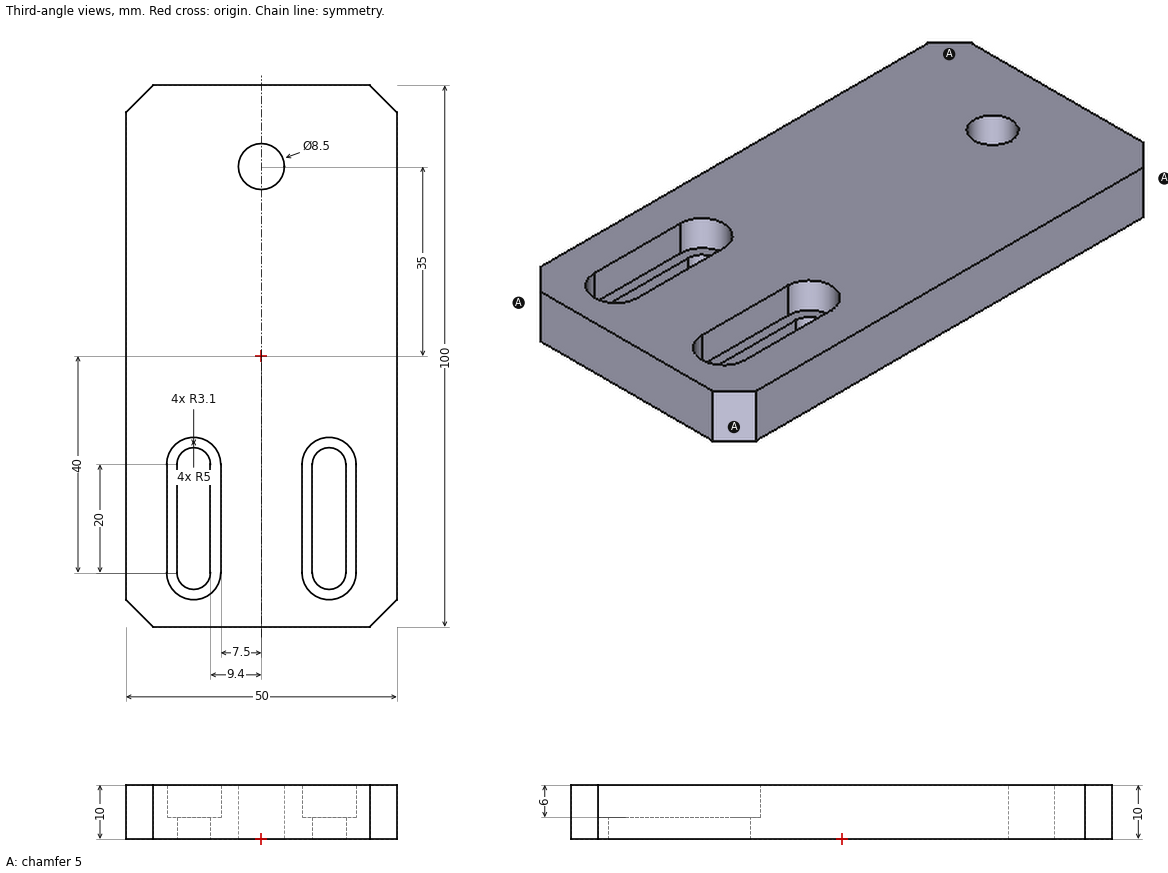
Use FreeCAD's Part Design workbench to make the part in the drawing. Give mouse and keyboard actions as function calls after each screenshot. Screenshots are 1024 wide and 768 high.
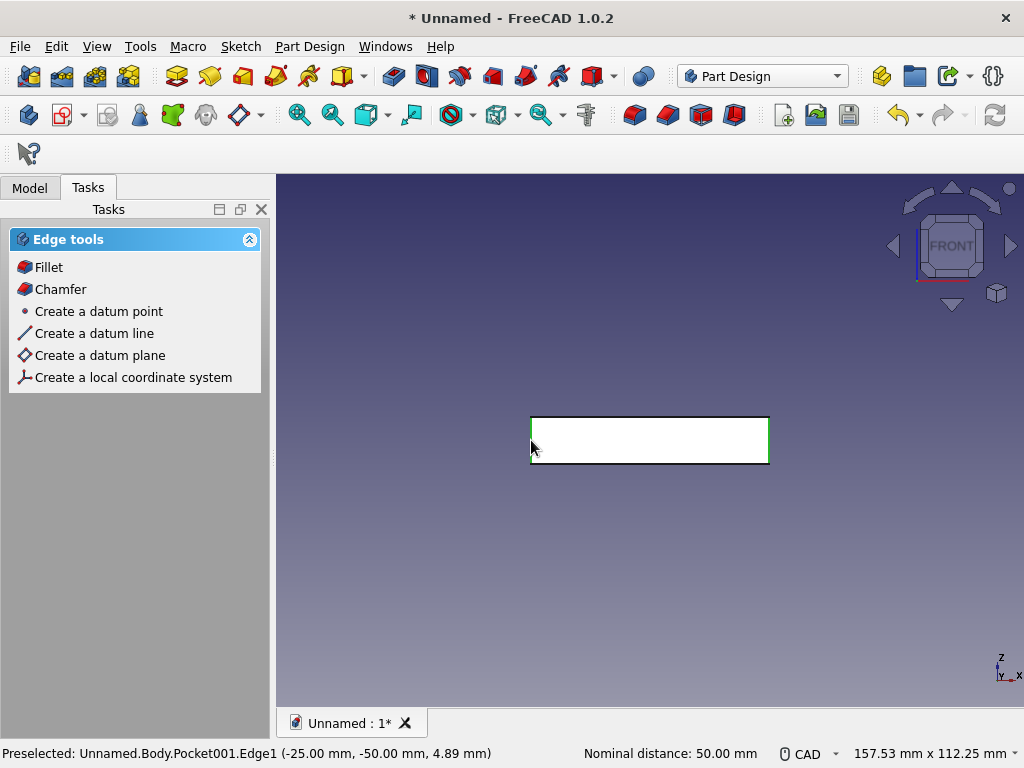
key(3)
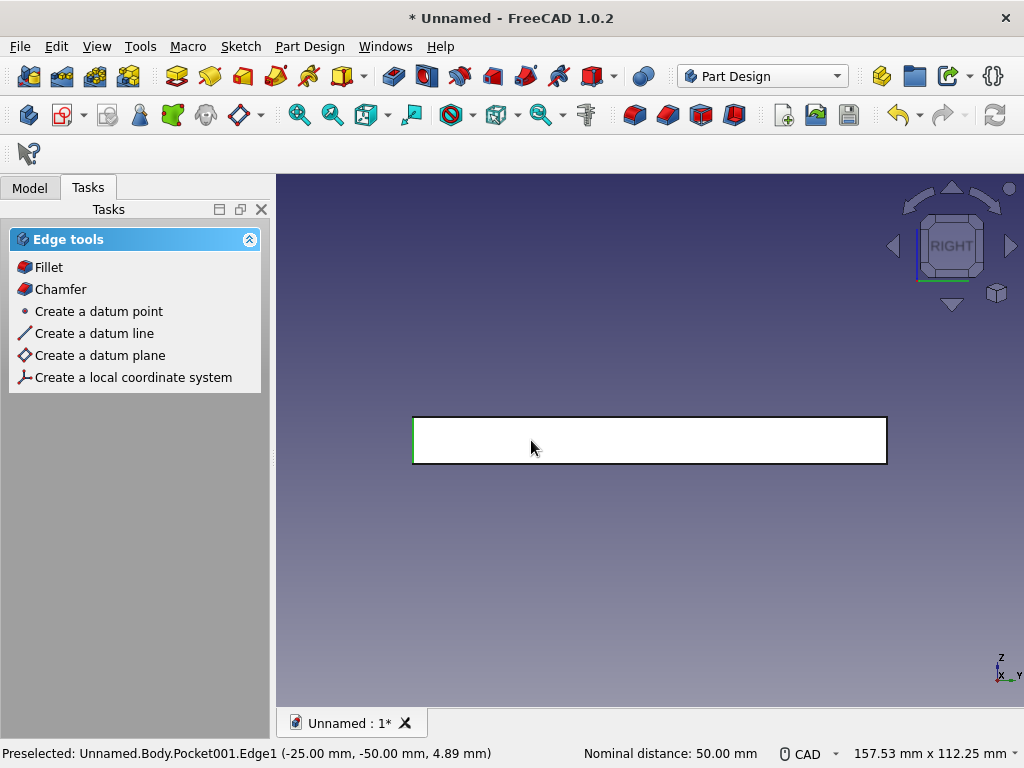
click(887, 439, ctrl)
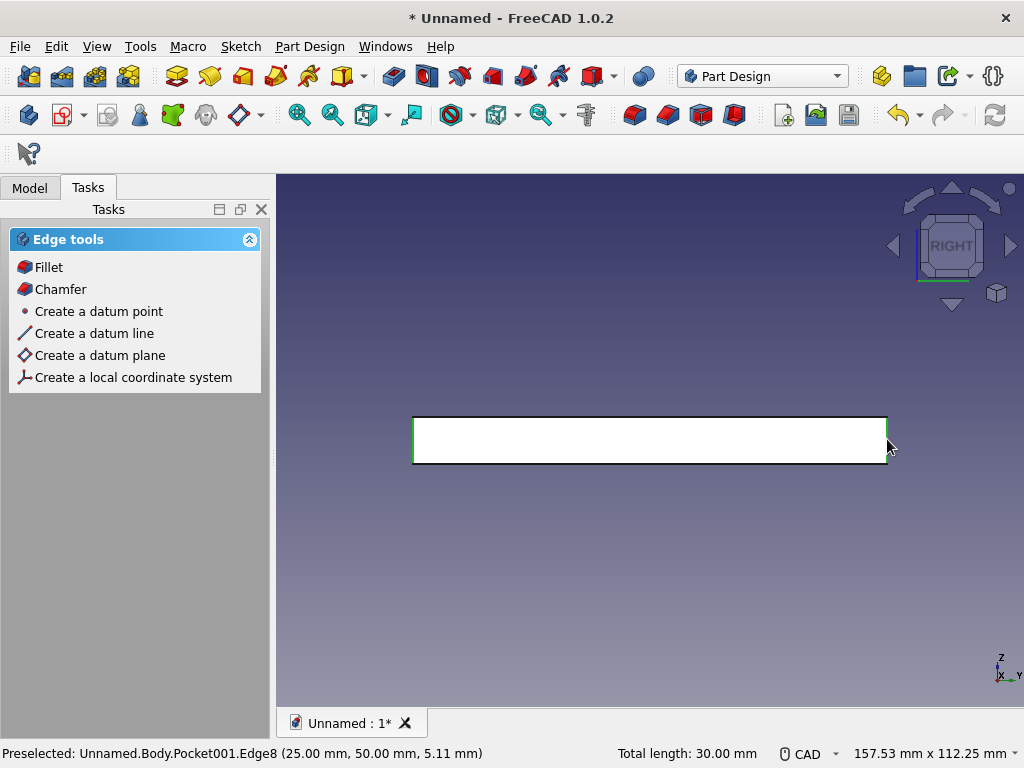
key(5)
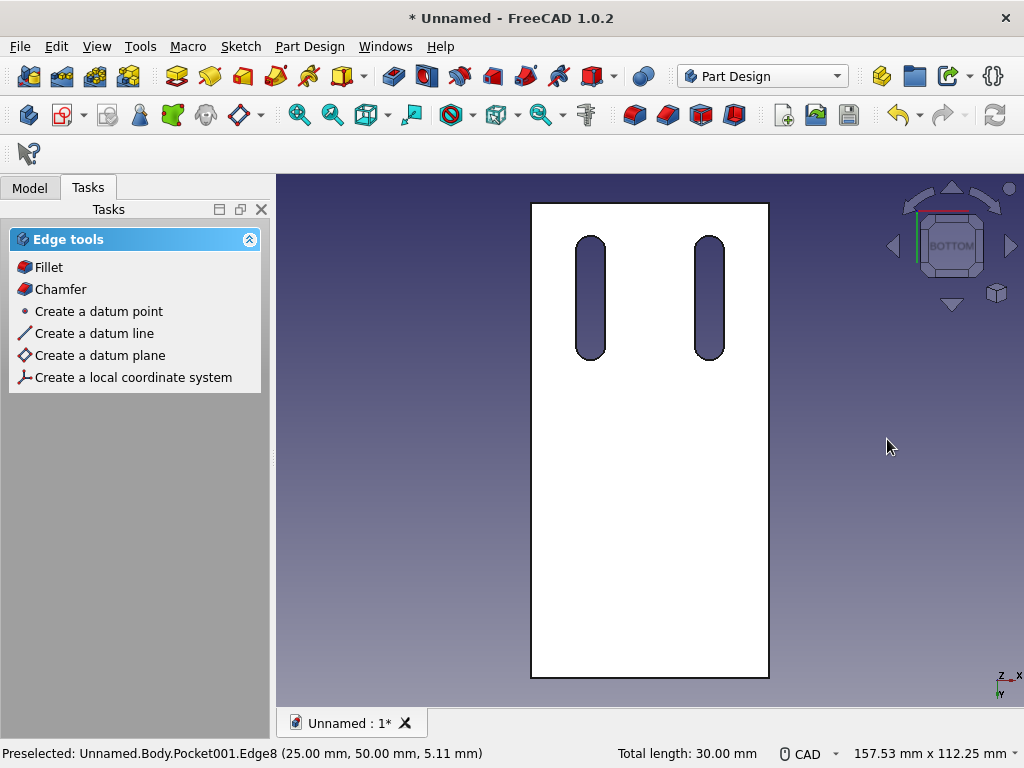
key(4)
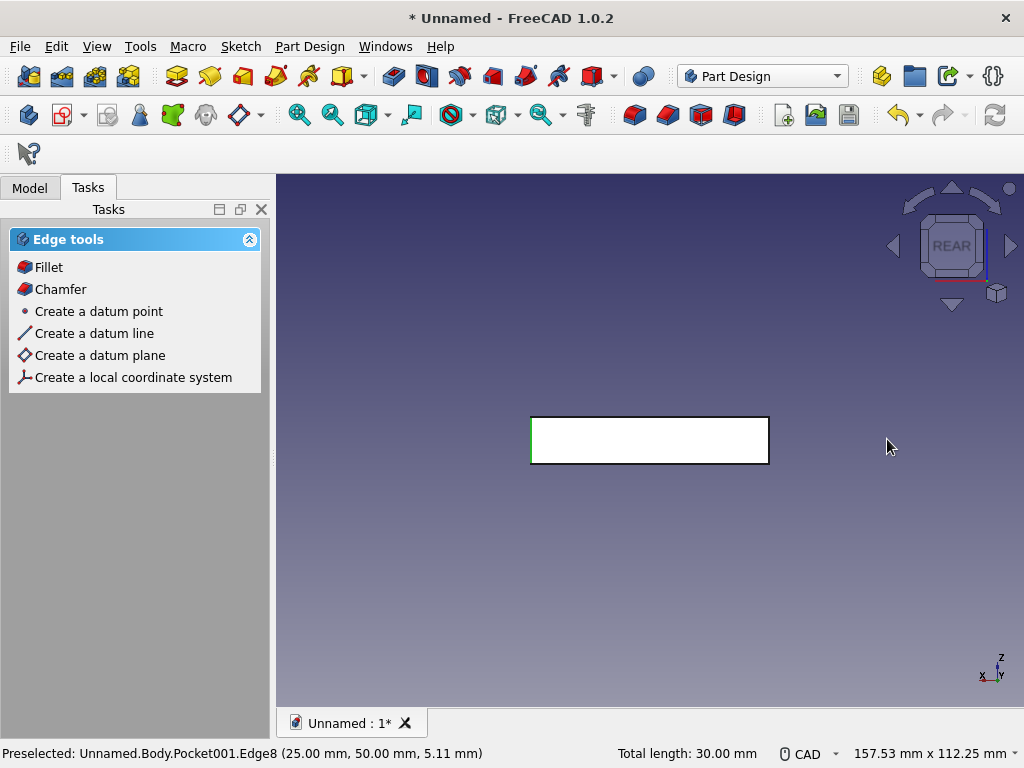
click(300, 116)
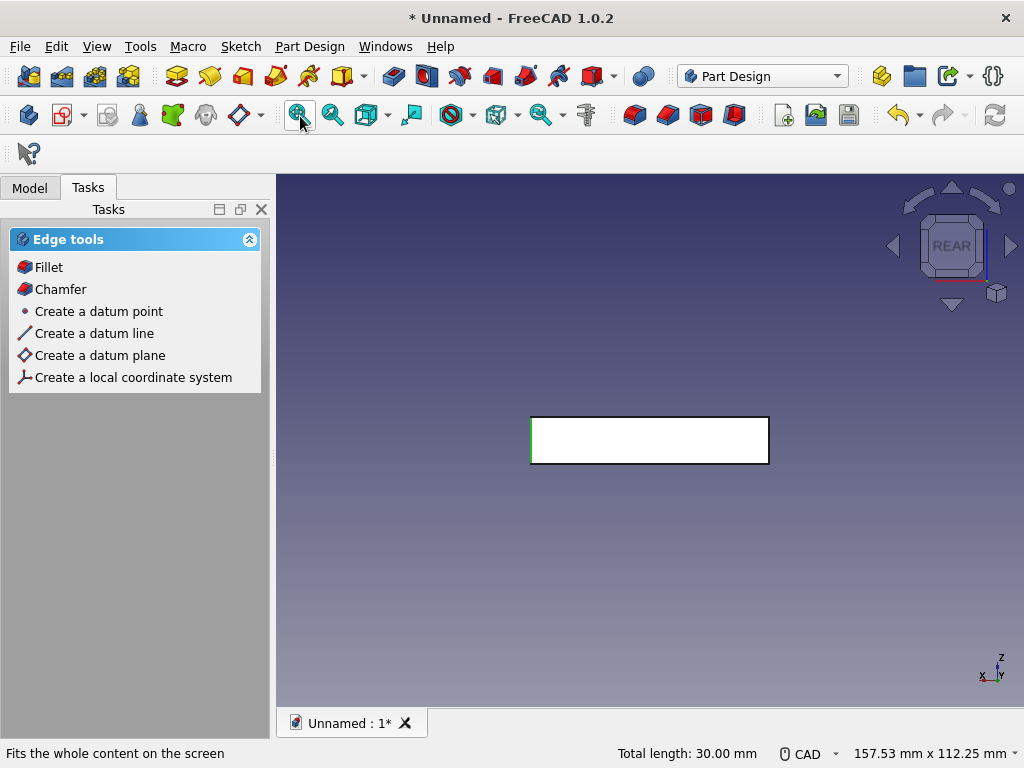
click(769, 440, ctrl)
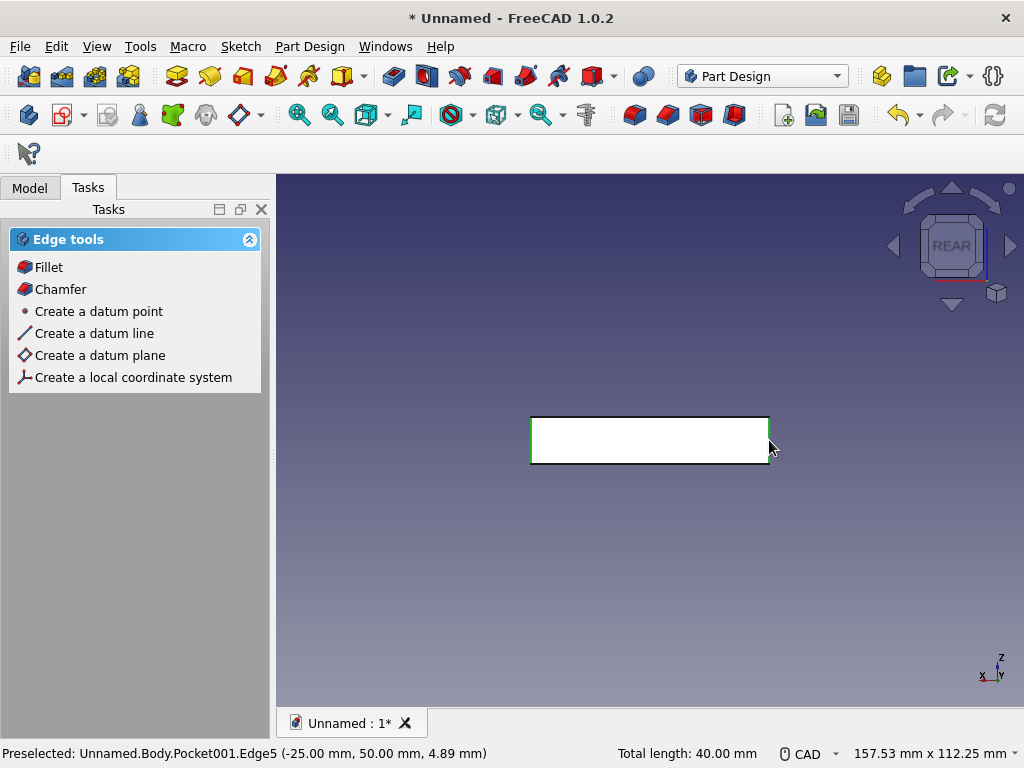
click(668, 116)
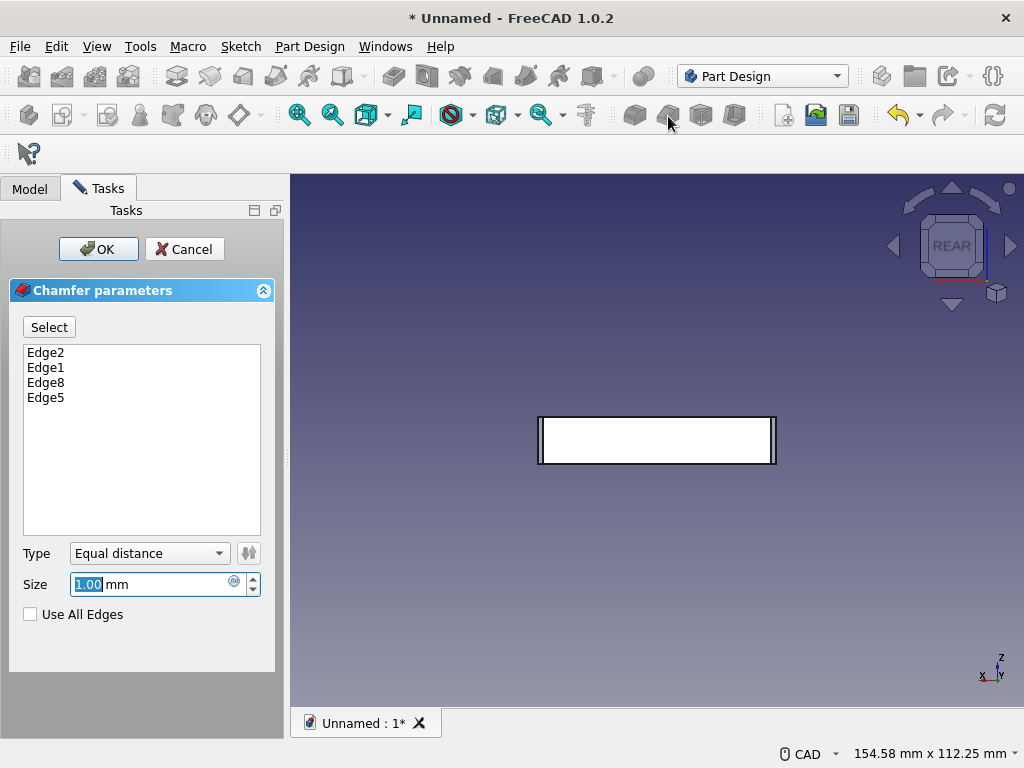
text(5)
key(Tab)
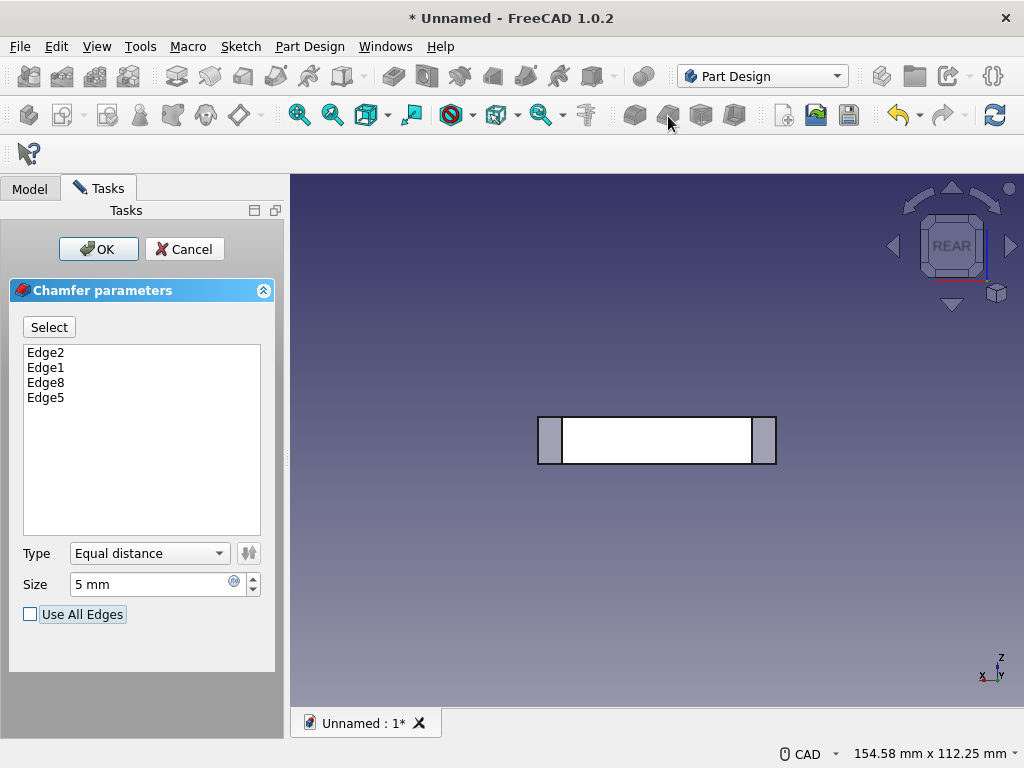
click(99, 249)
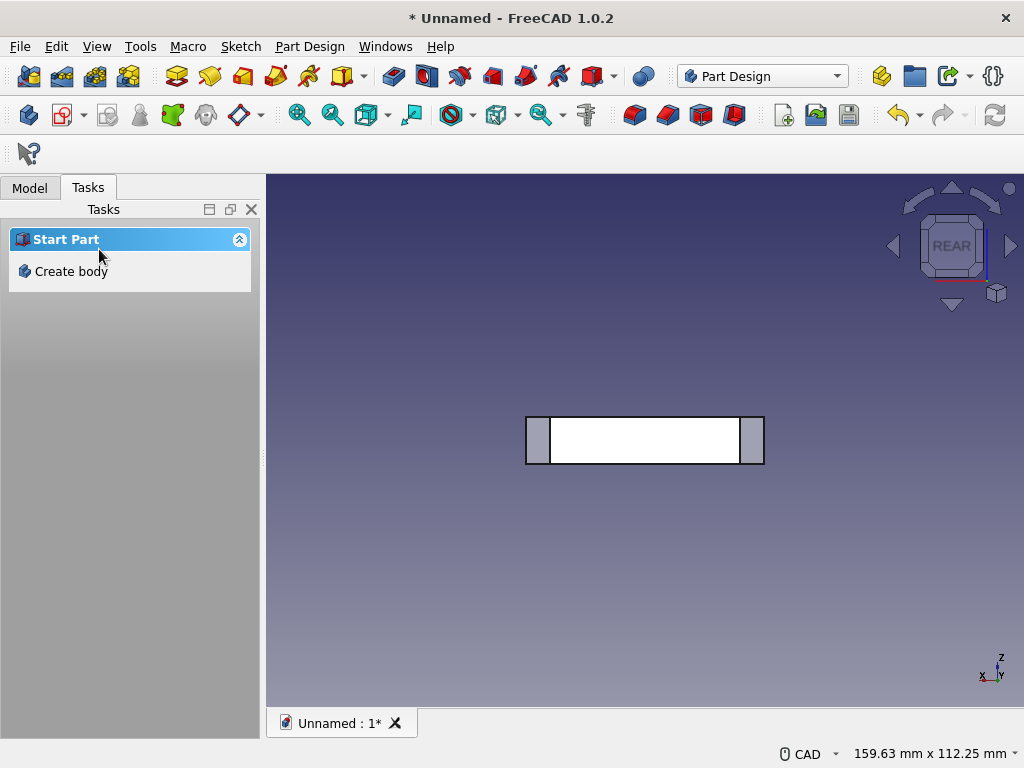
click(300, 116)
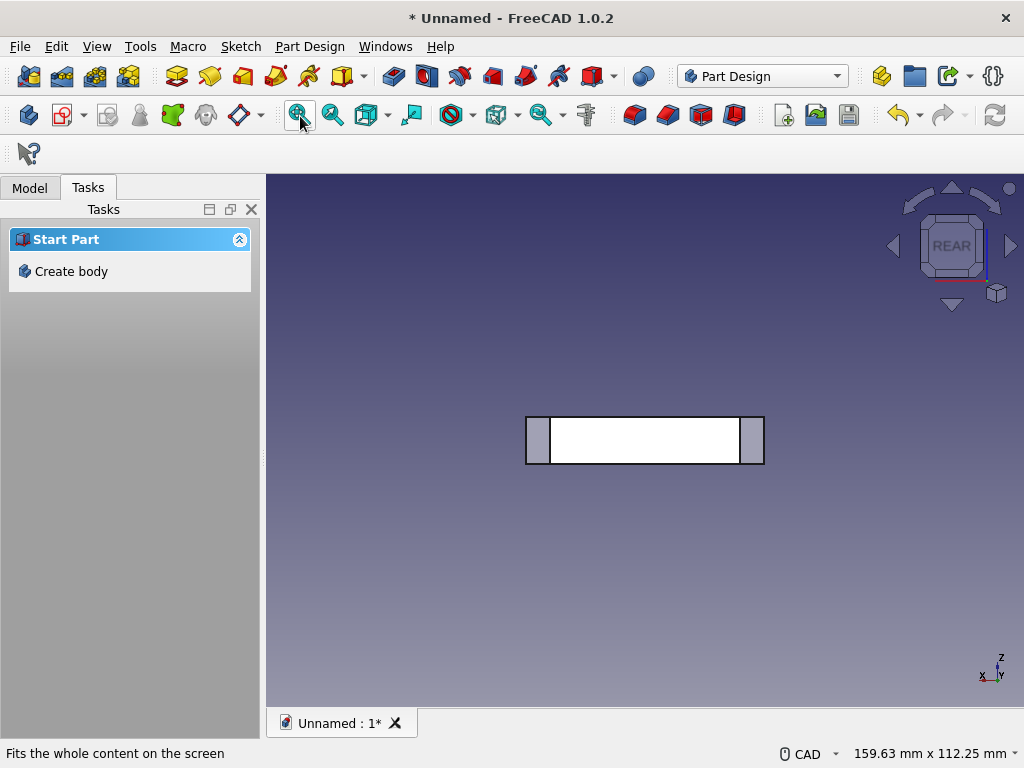
key(0)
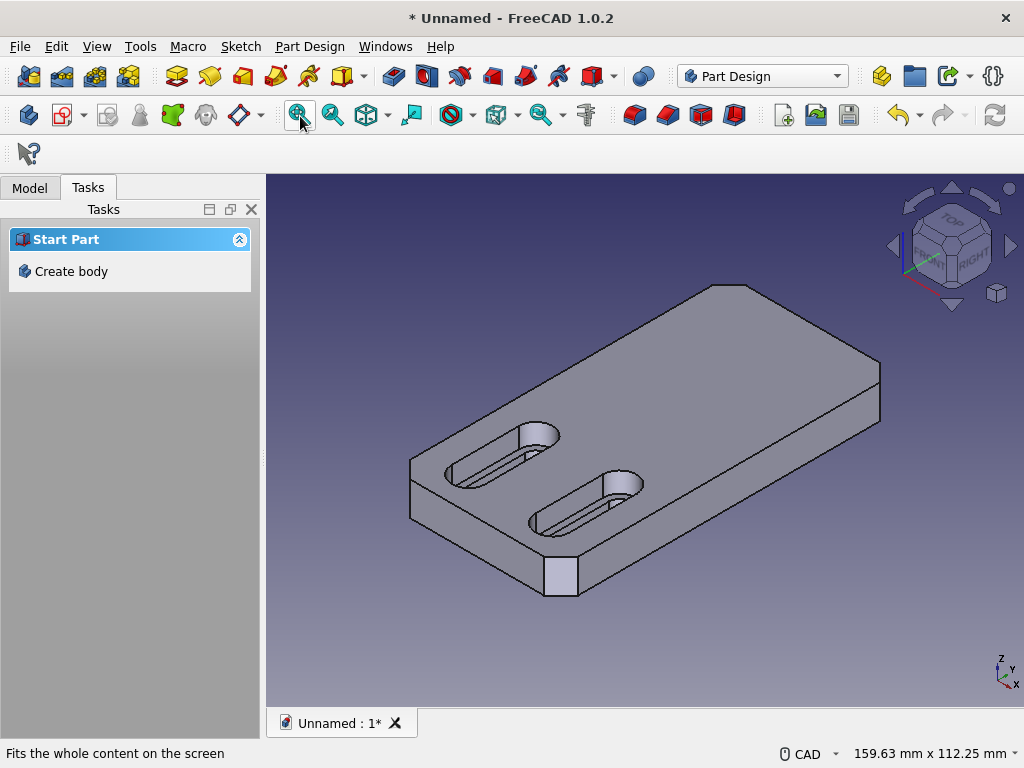
click(693, 392)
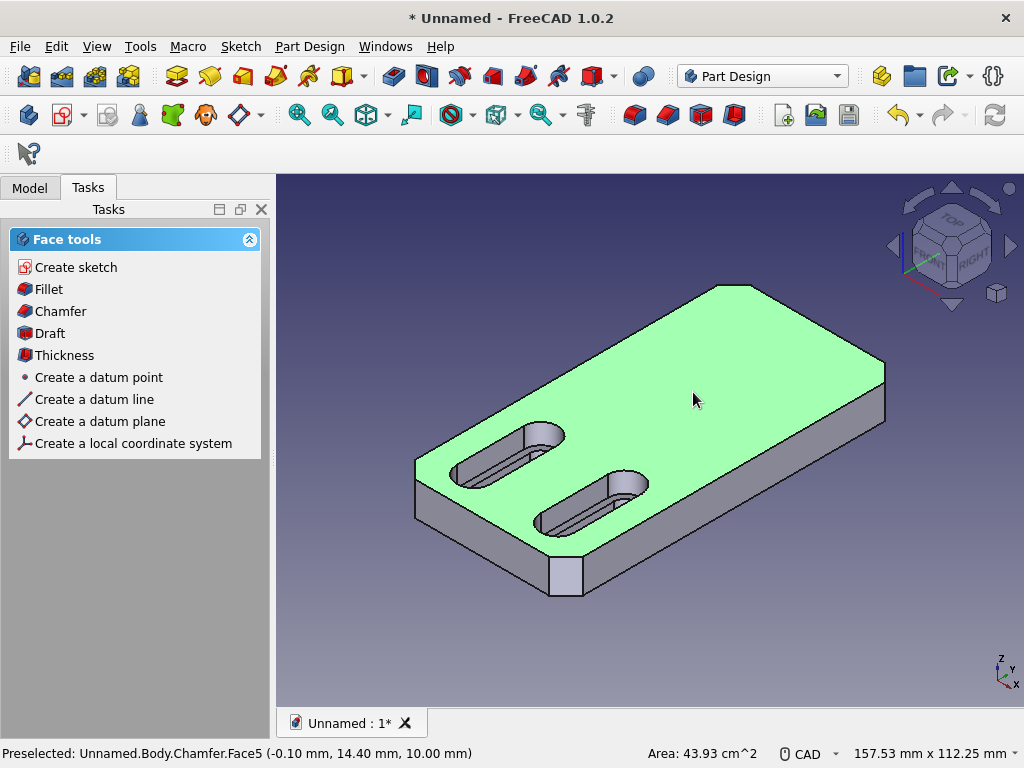
click(62, 116)